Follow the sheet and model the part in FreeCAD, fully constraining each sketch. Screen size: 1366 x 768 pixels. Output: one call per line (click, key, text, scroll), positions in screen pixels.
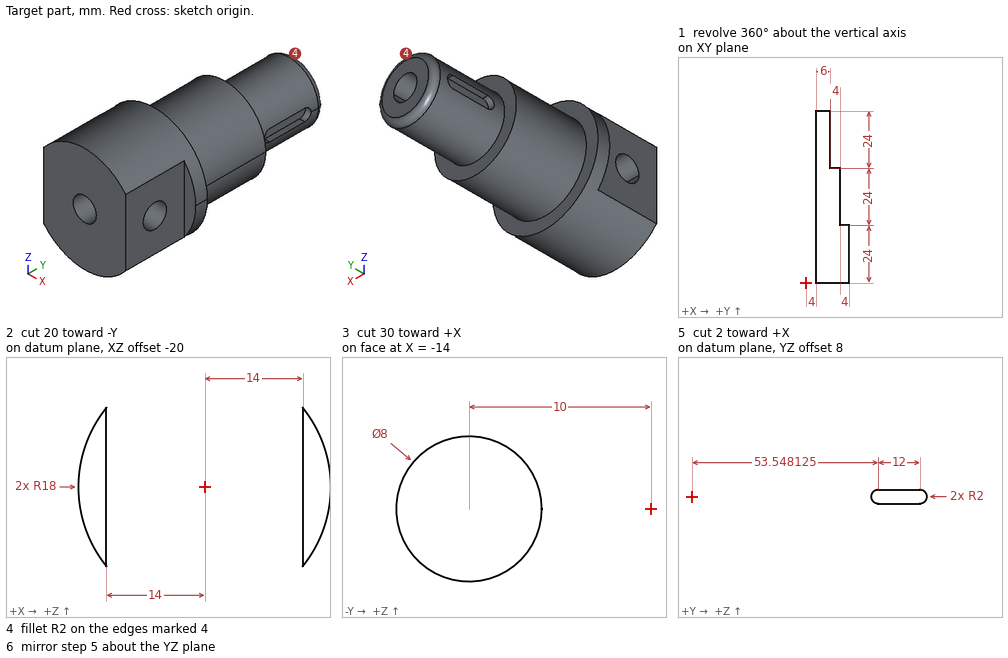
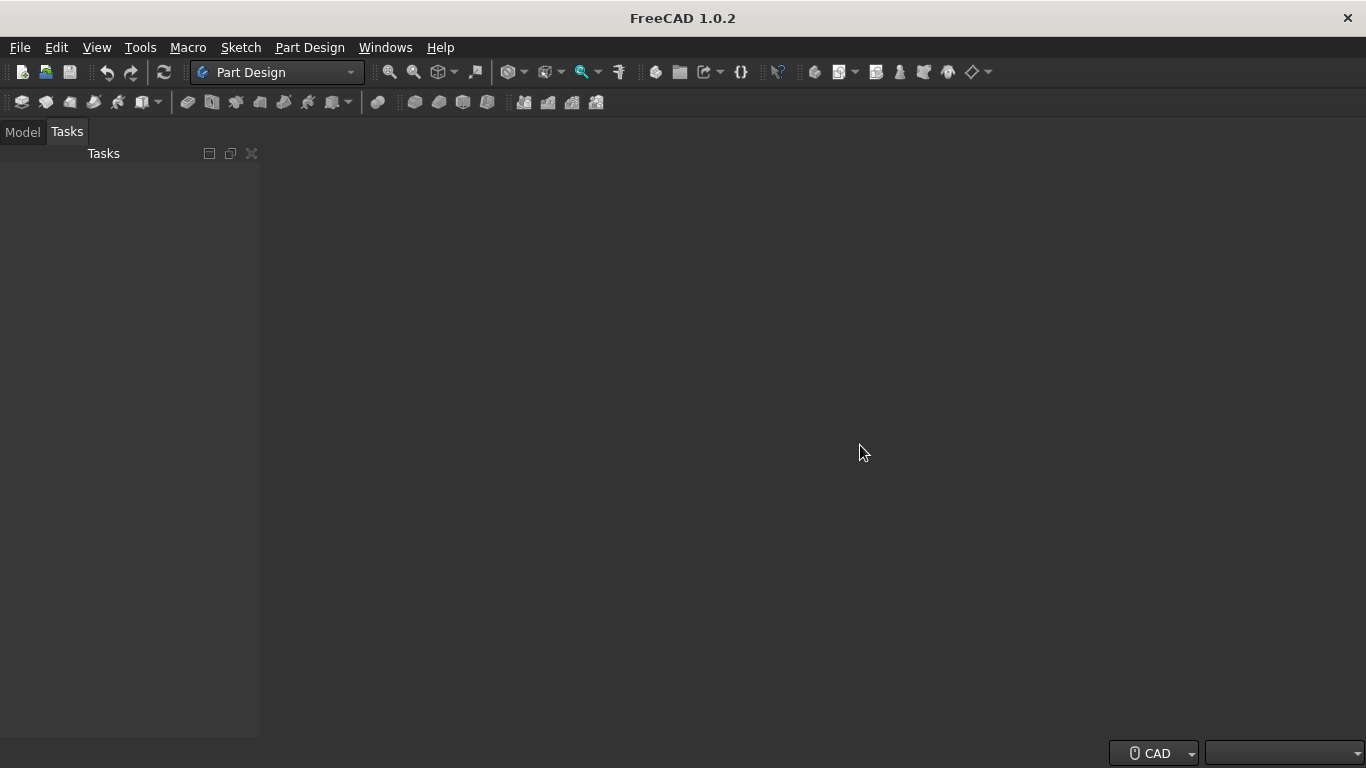
click(22, 72)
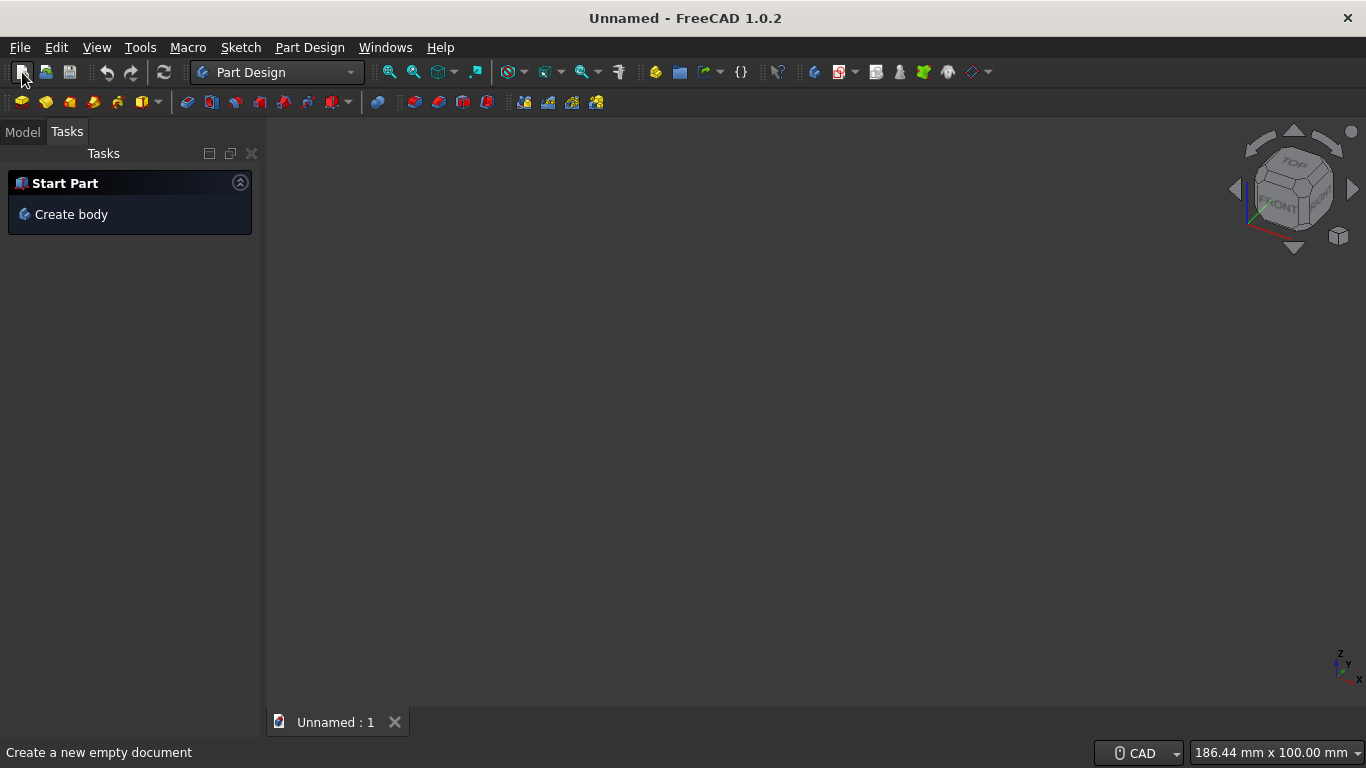
click(840, 72)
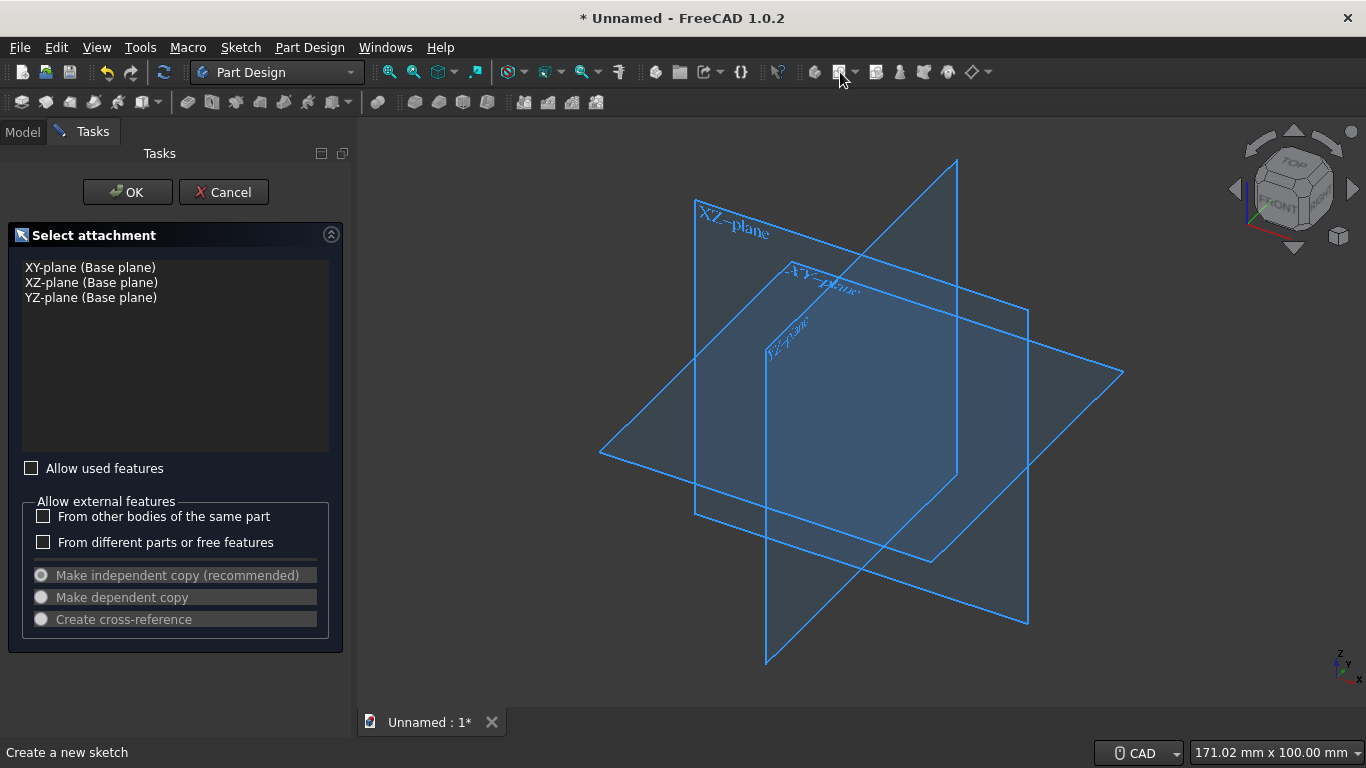
click(82, 268)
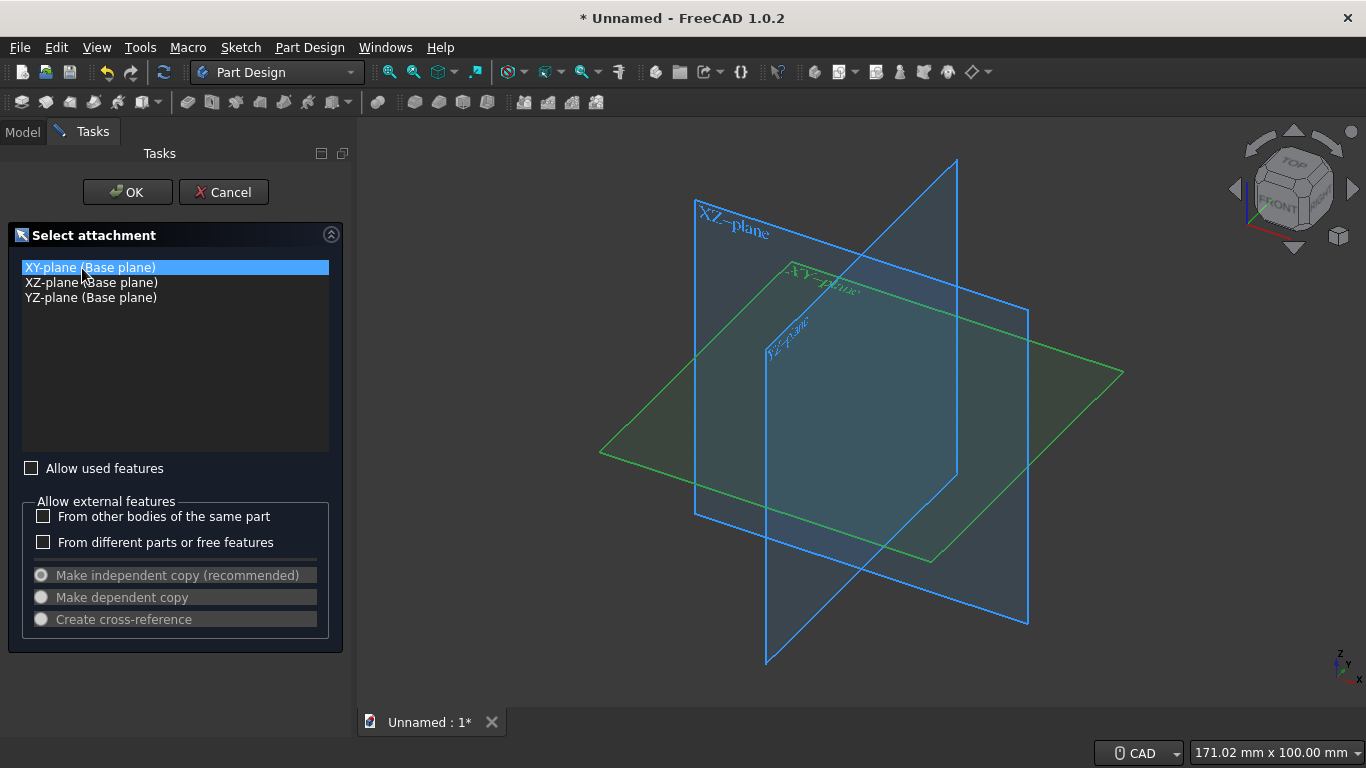
click(128, 192)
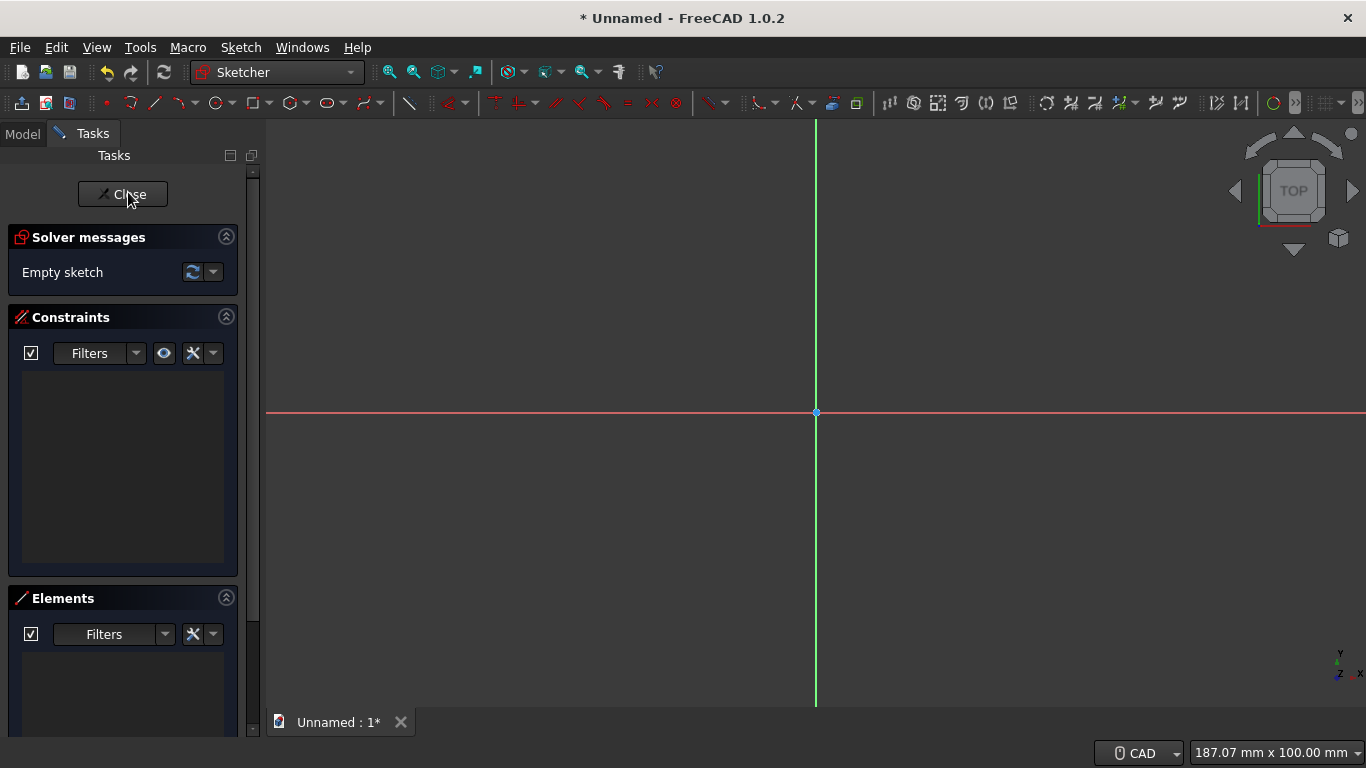
scroll(501, 679, down, 2)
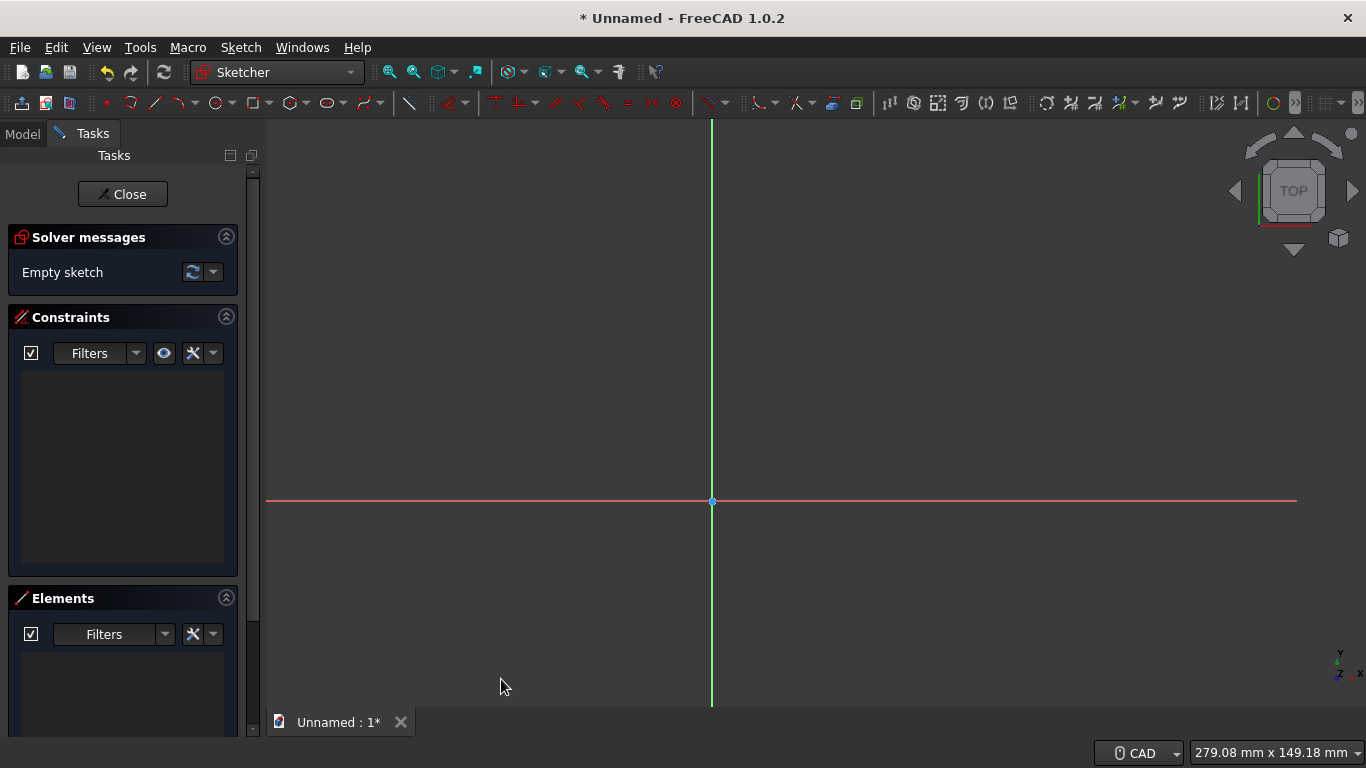
click(132, 104)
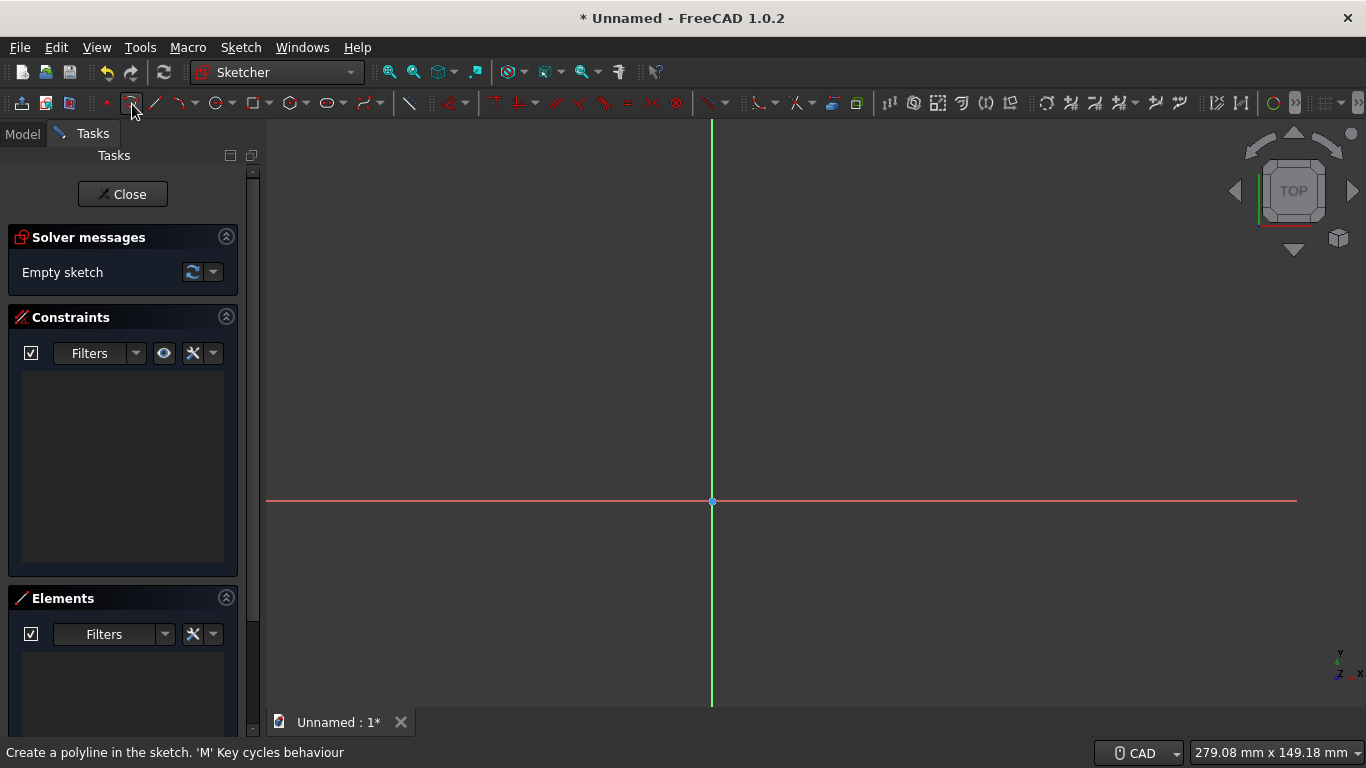
click(728, 501)
click(783, 492)
click(783, 406)
click(767, 406)
click(767, 312)
click(752, 312)
click(752, 217)
click(728, 217)
click(728, 501)
key(Escape)
key(Escape)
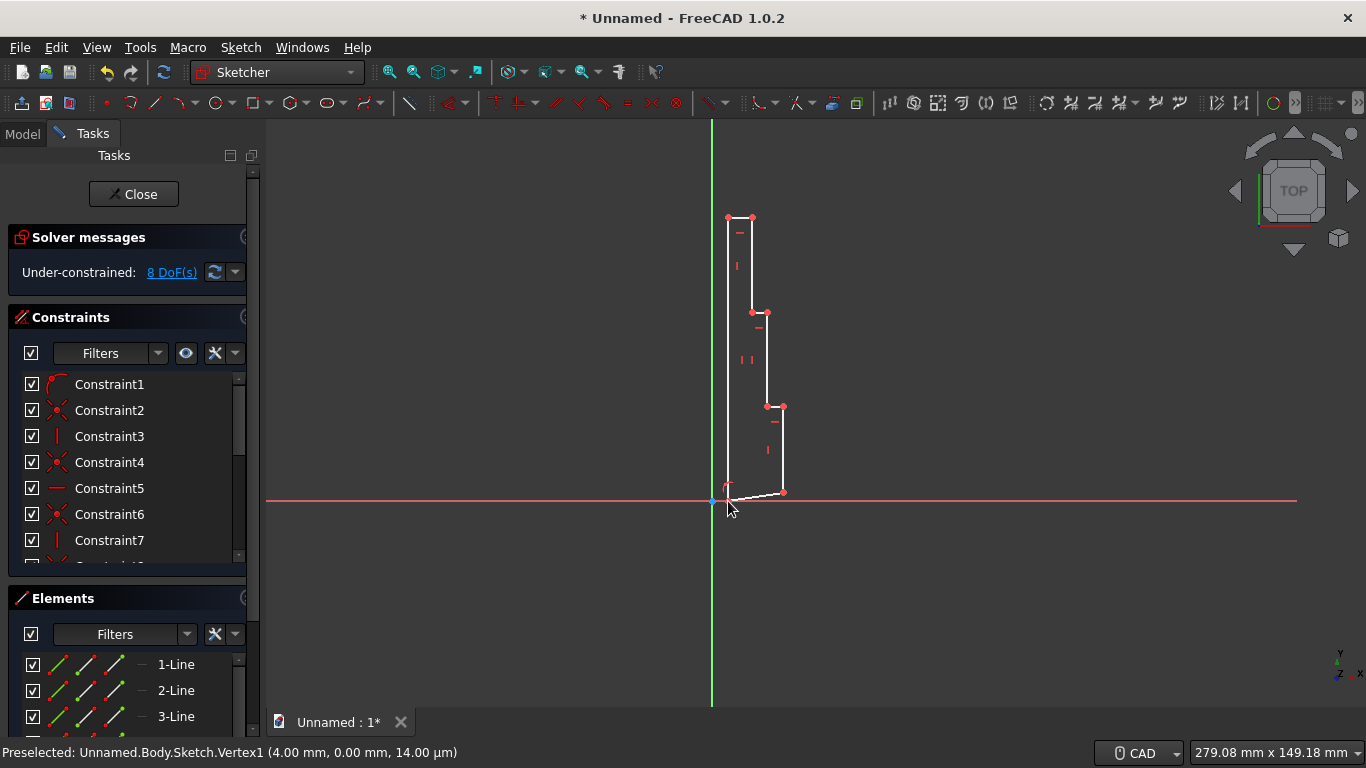
click(744, 499)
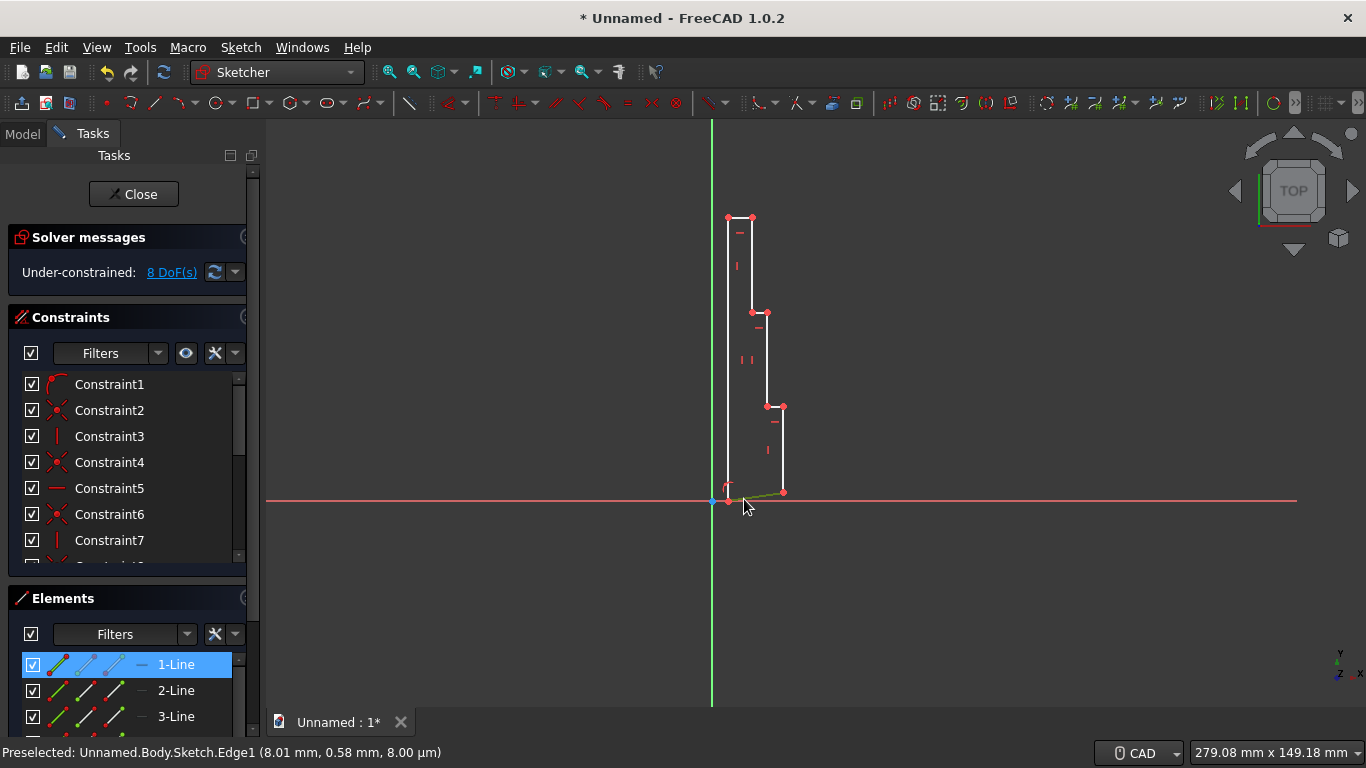
key(h)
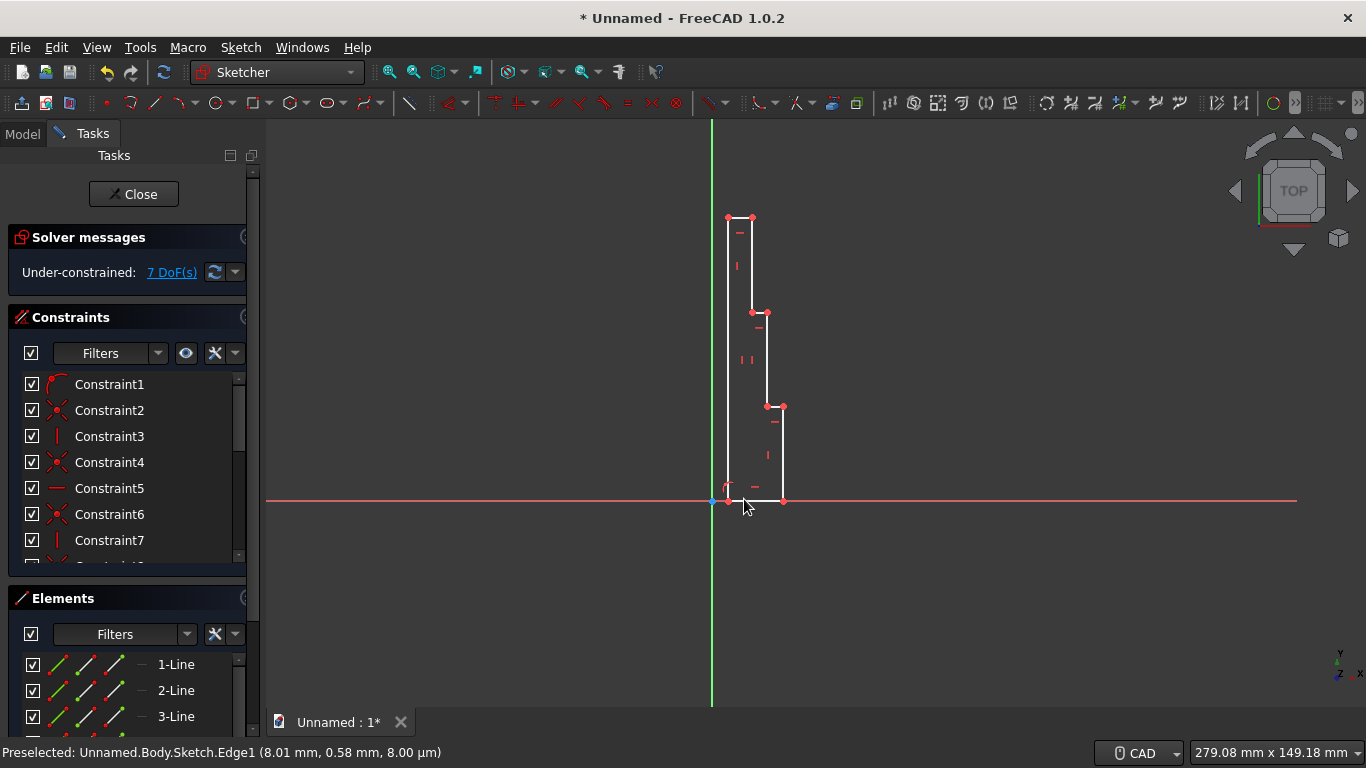
click(448, 104)